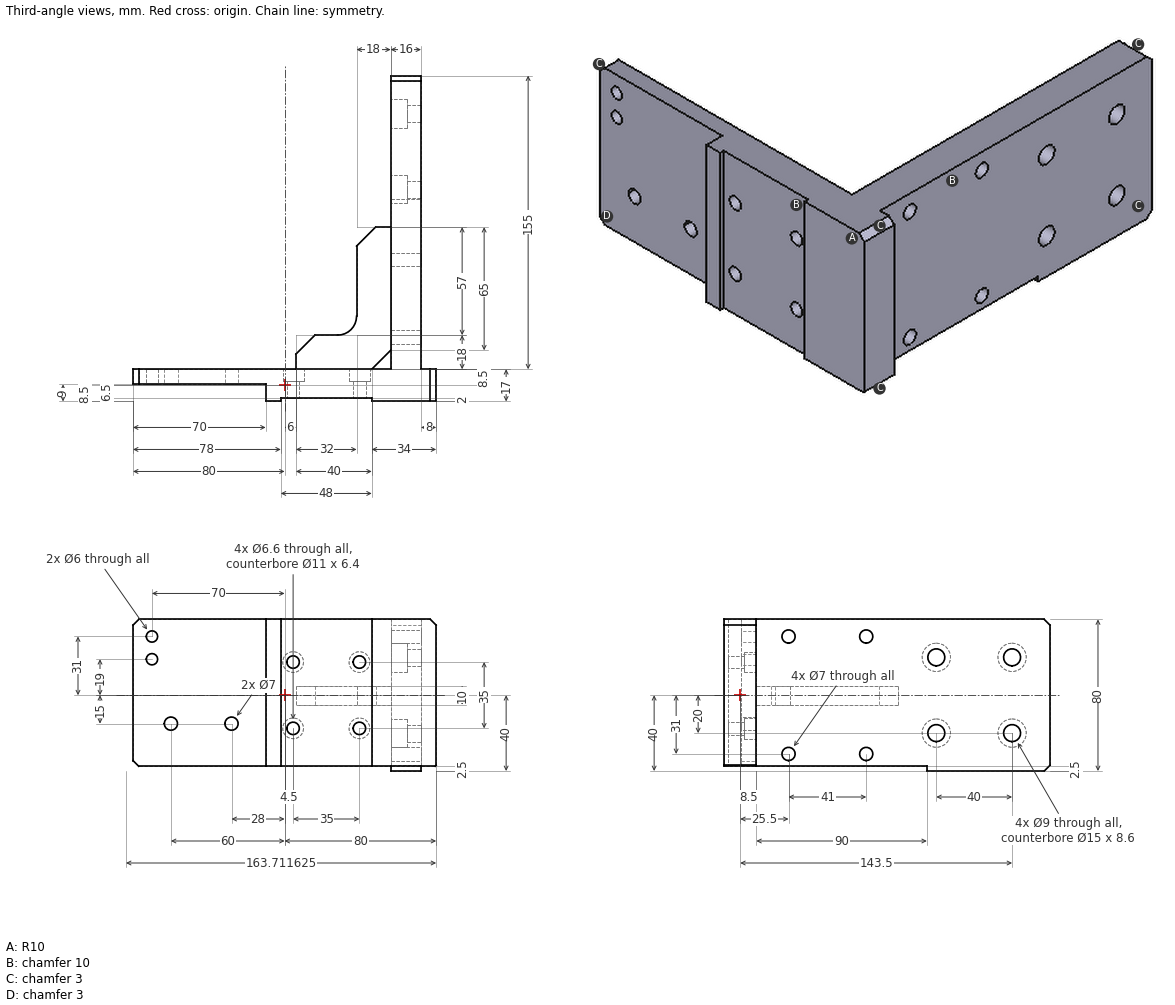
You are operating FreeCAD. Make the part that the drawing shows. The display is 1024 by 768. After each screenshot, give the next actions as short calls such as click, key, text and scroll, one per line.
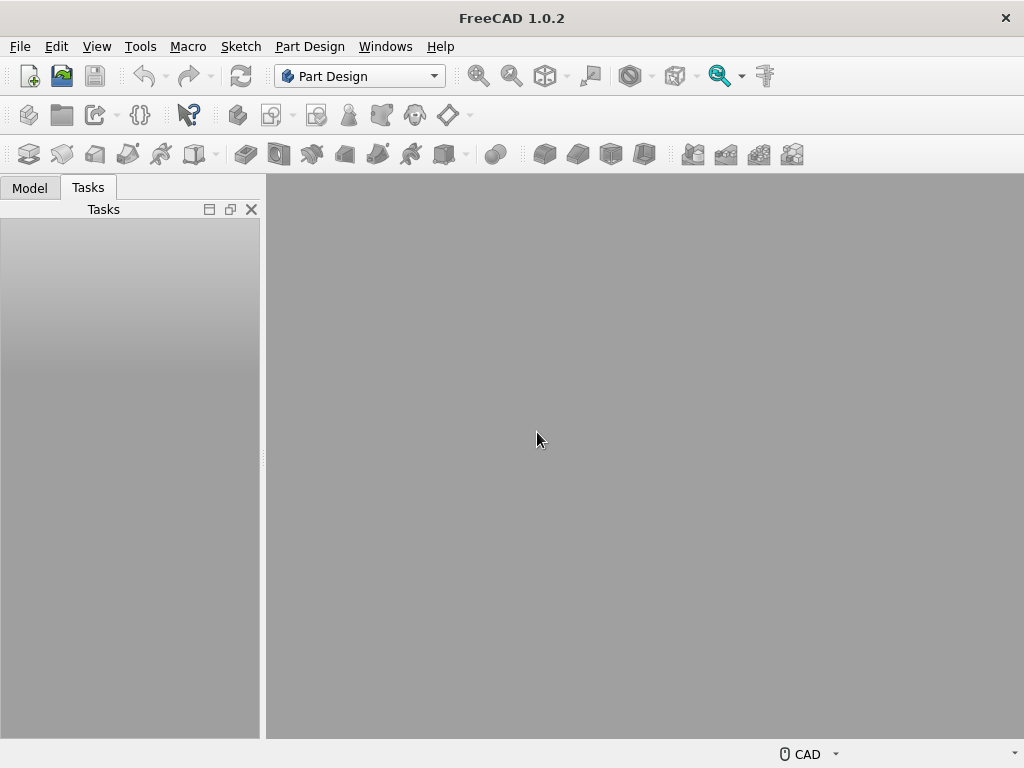
click(29, 76)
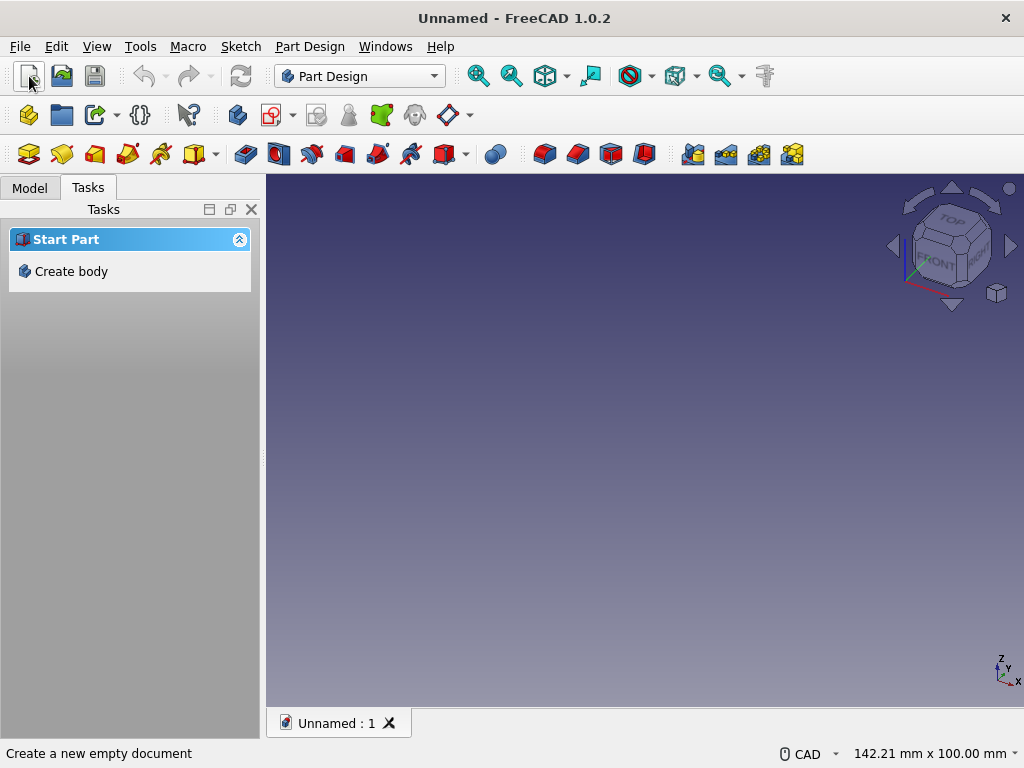
click(270, 116)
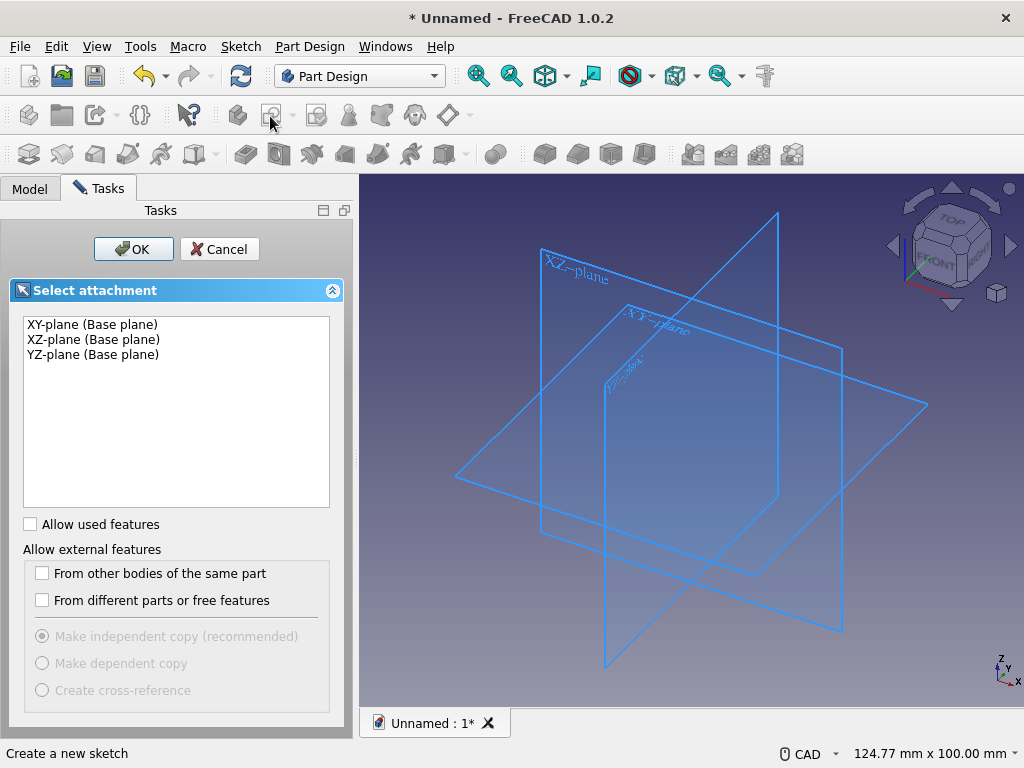
click(84, 324)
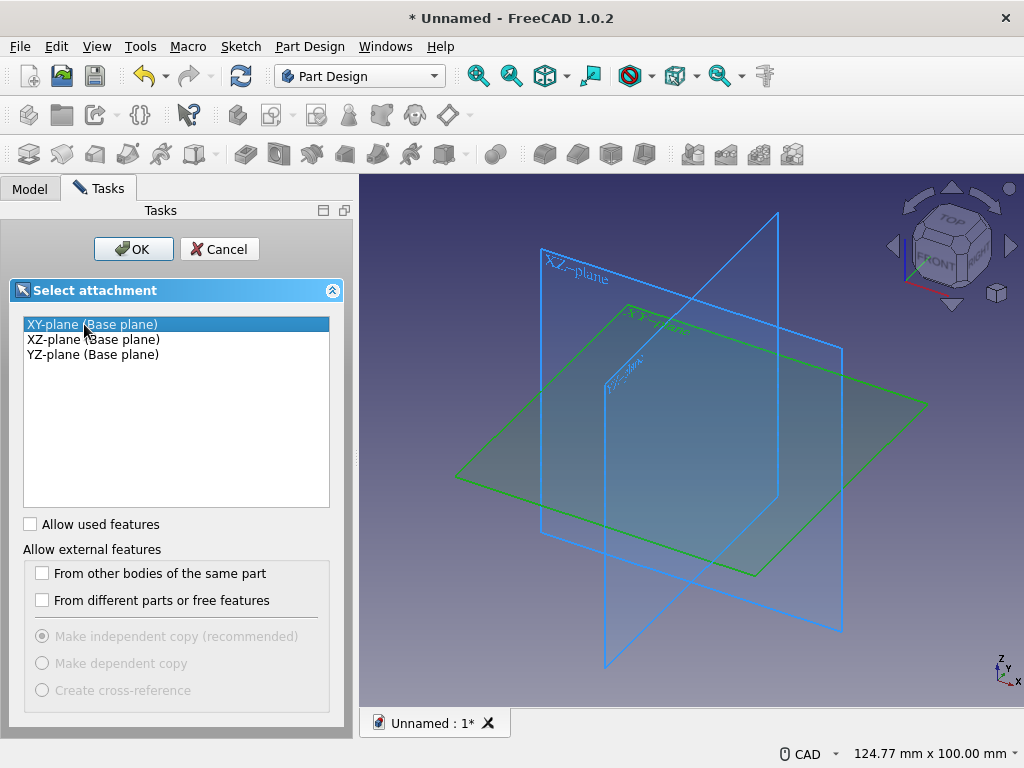
click(134, 249)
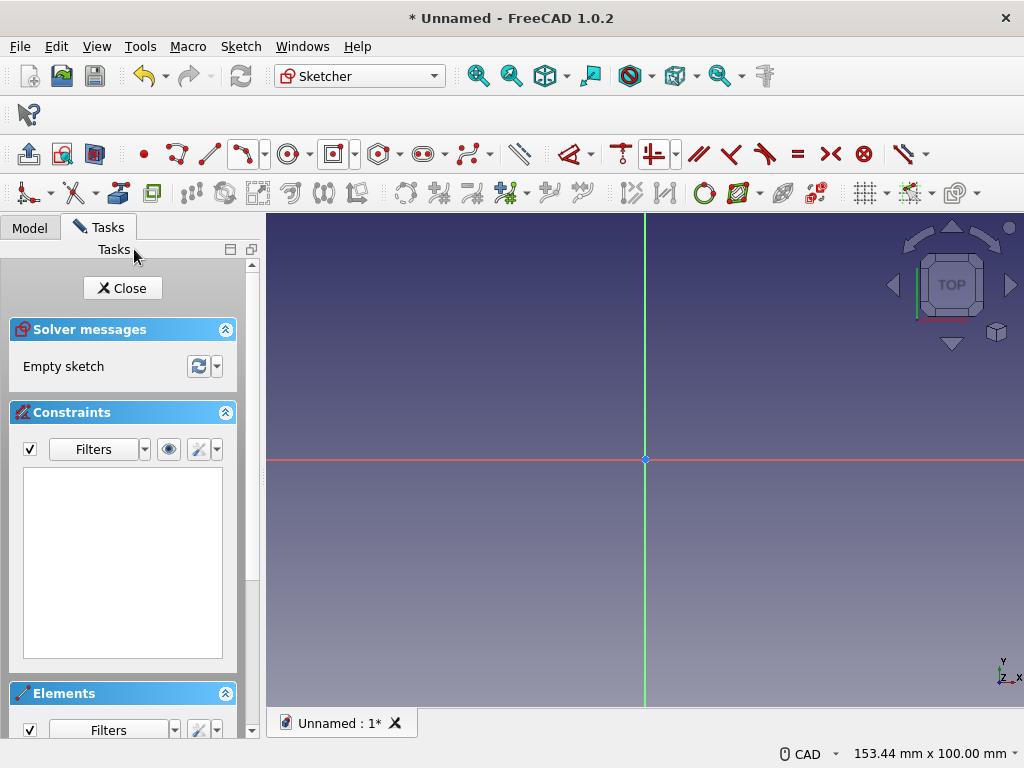
scroll(537, 679, down, 5)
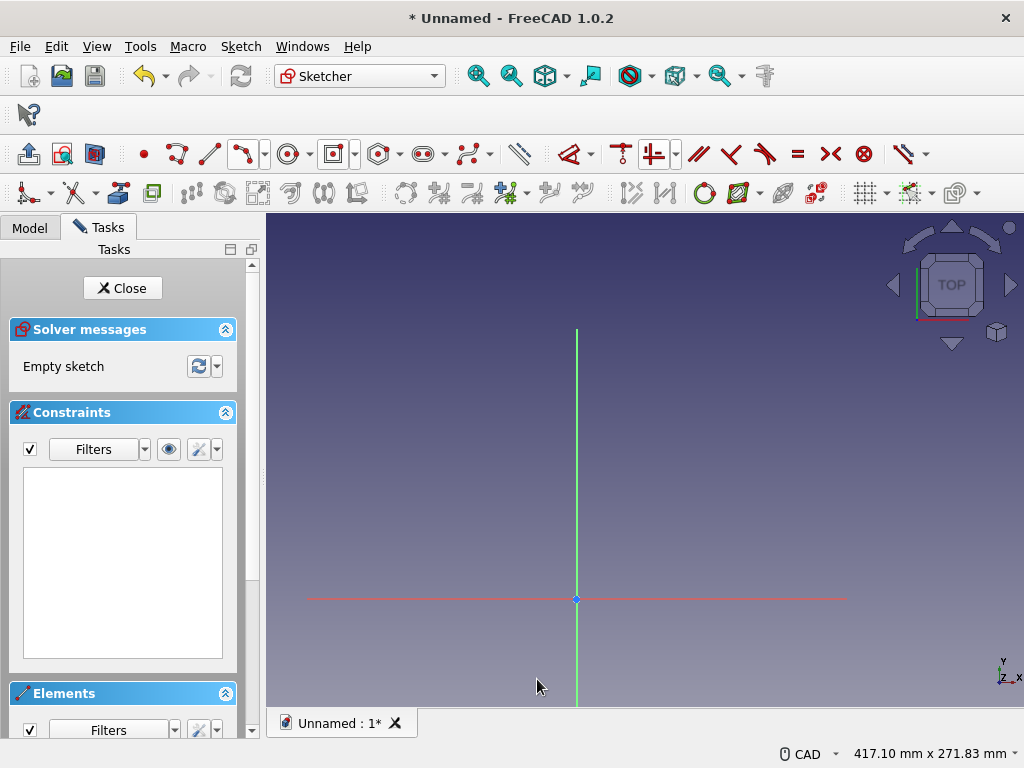
click(177, 154)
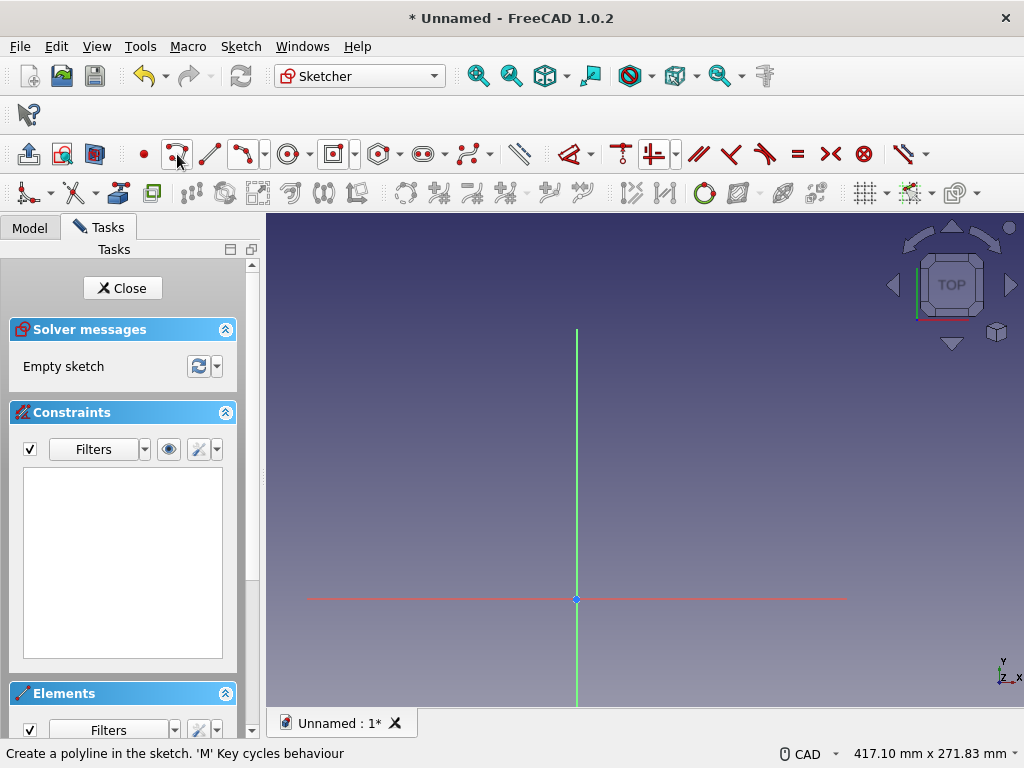
scroll(573, 611, up, 8)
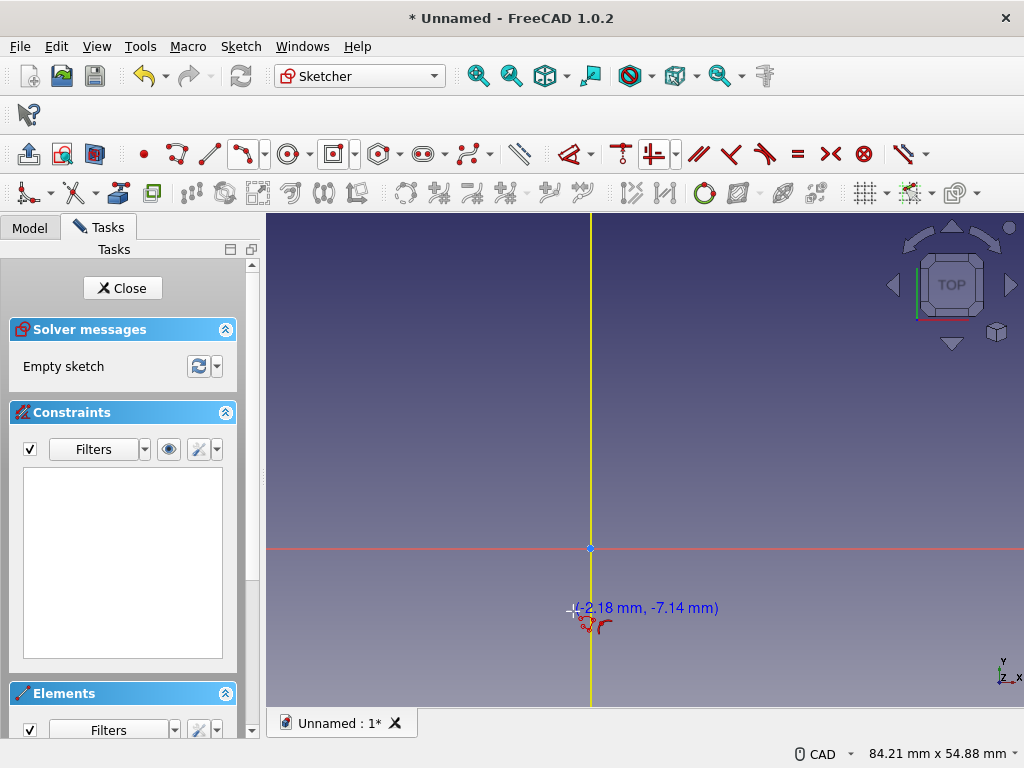
click(573, 607)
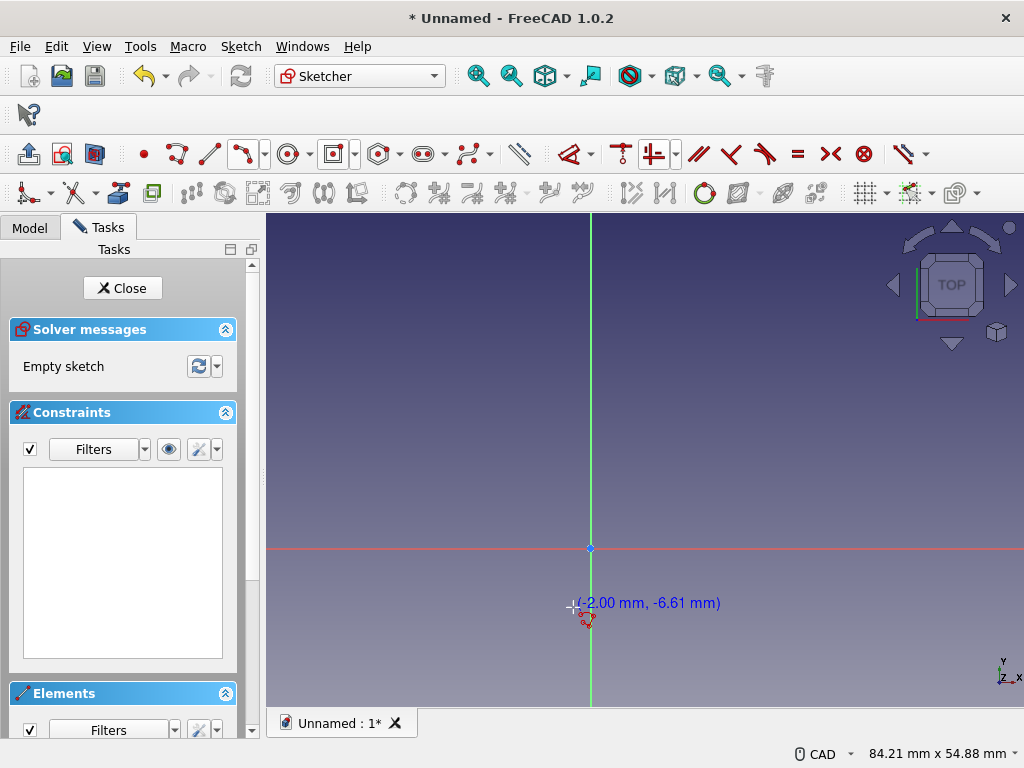
scroll(573, 614, down, 8)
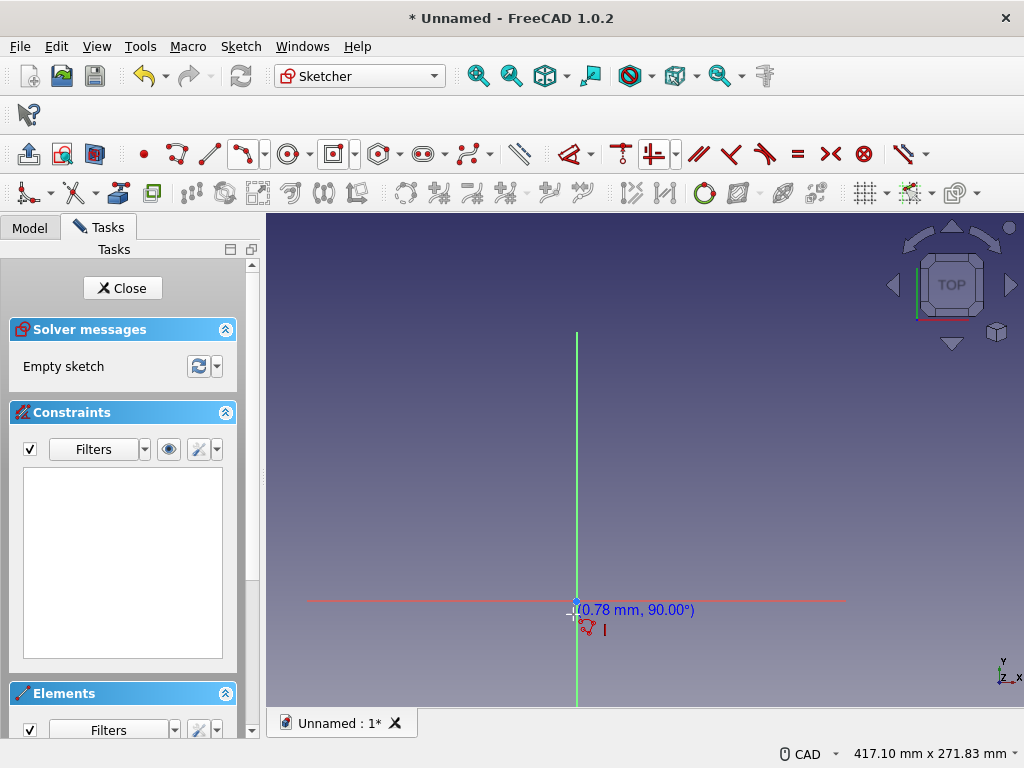
scroll(661, 613, up, 2)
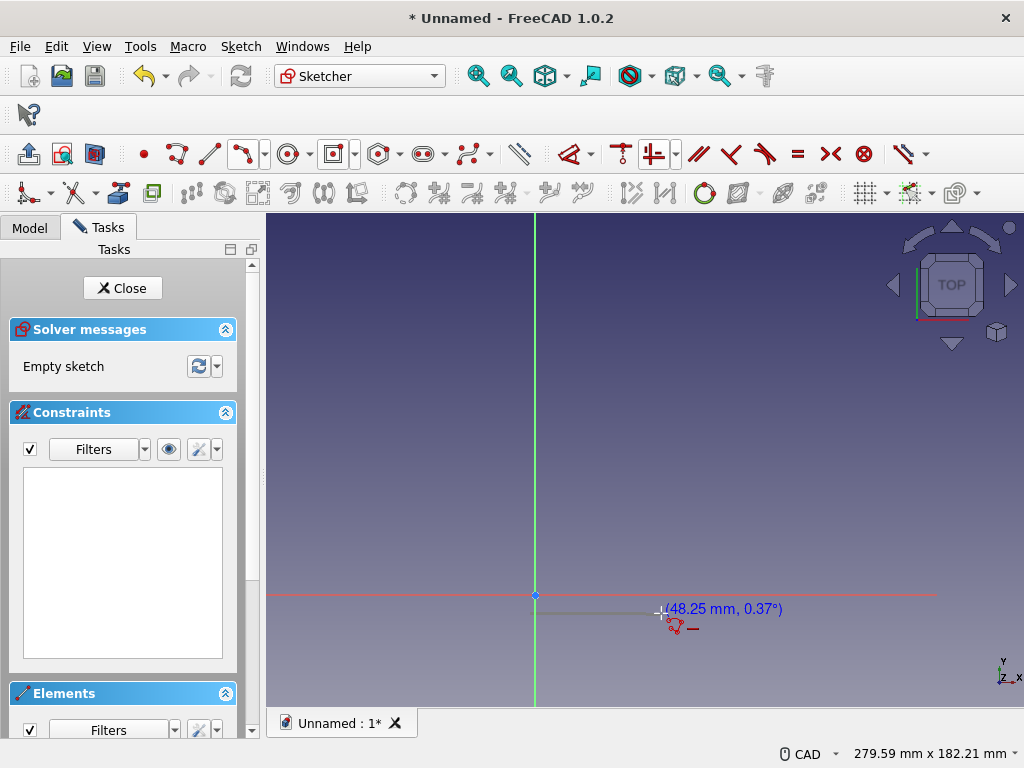
click(660, 613)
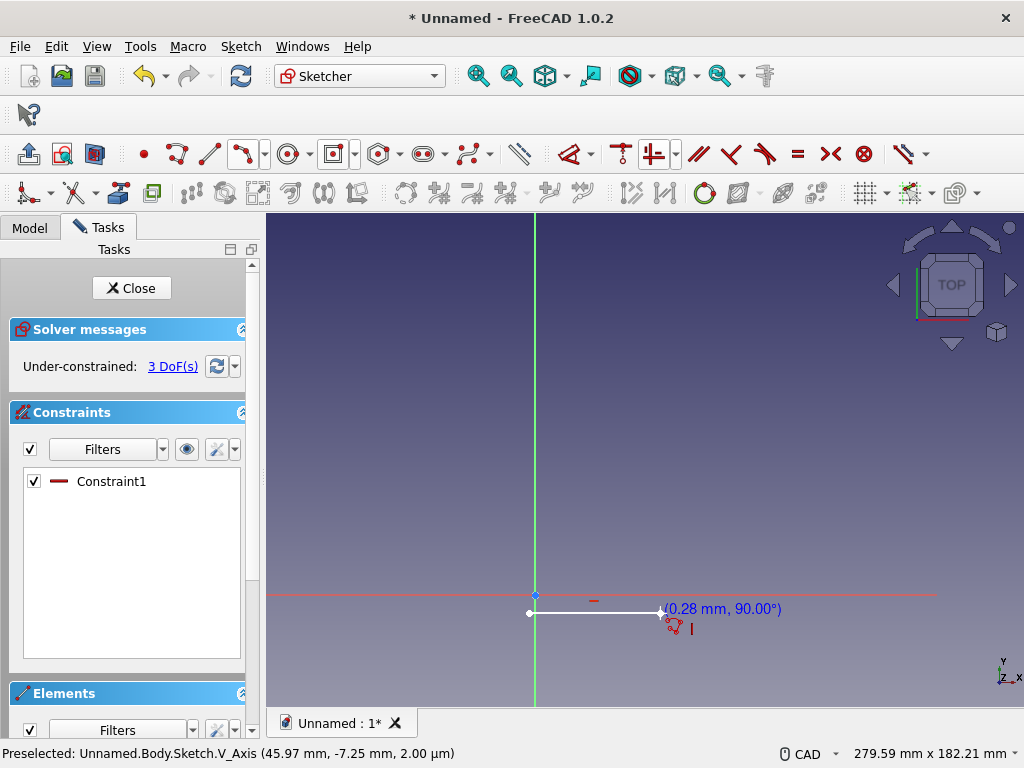
scroll(660, 618, up, 6)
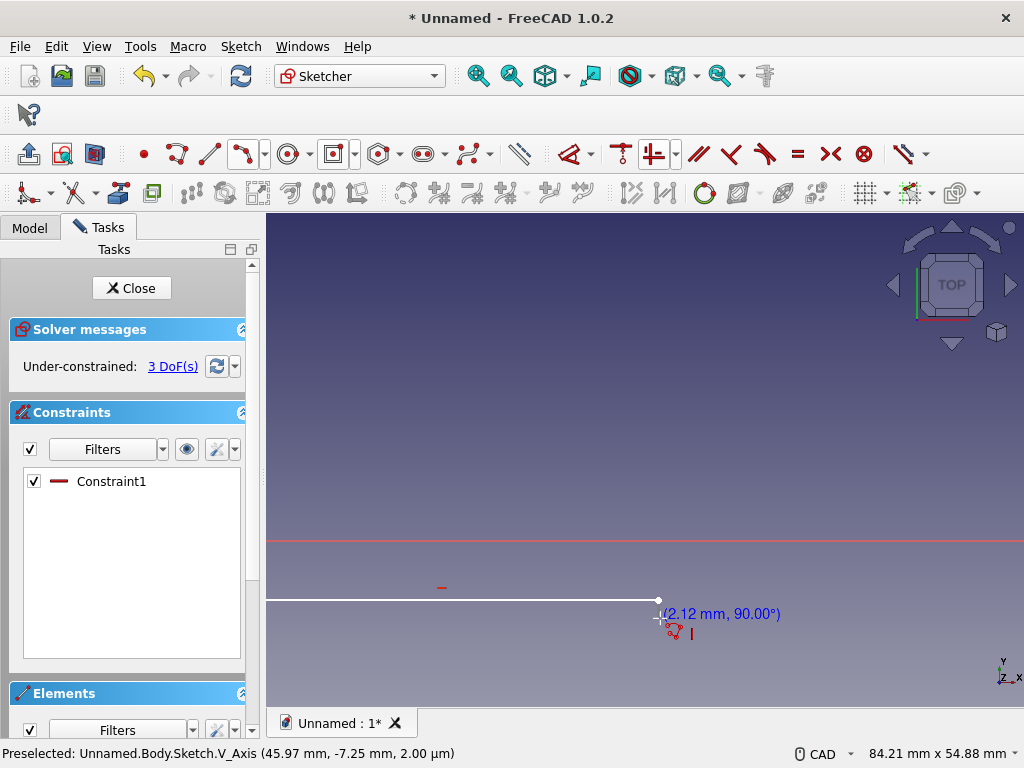
click(659, 617)